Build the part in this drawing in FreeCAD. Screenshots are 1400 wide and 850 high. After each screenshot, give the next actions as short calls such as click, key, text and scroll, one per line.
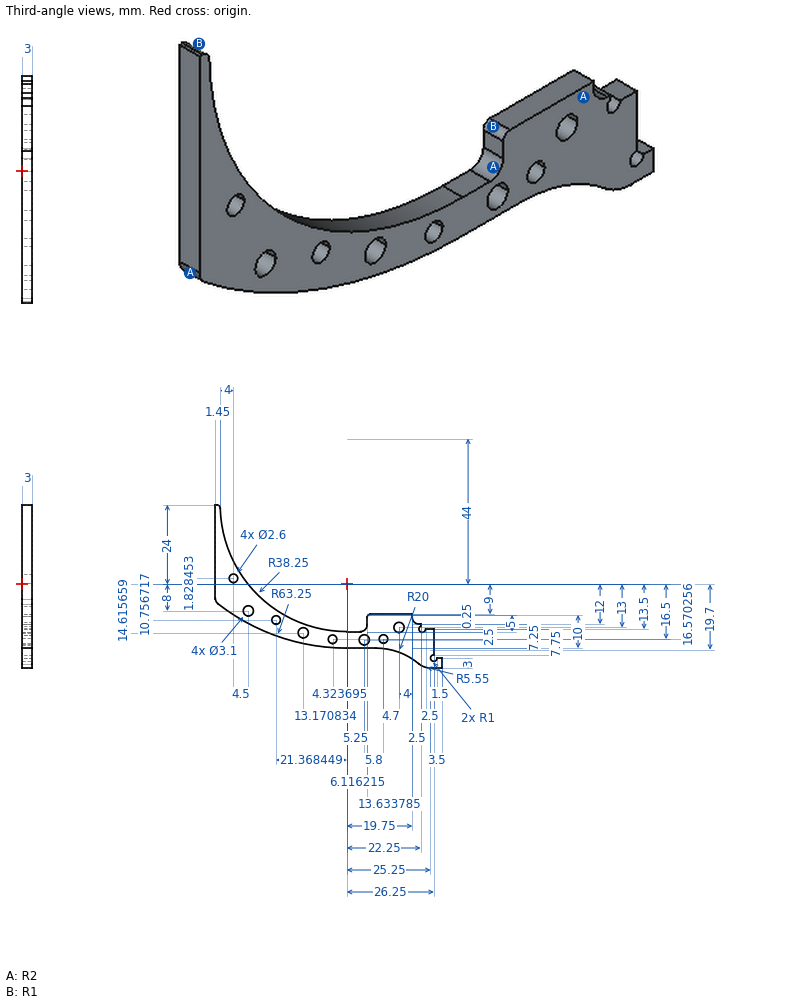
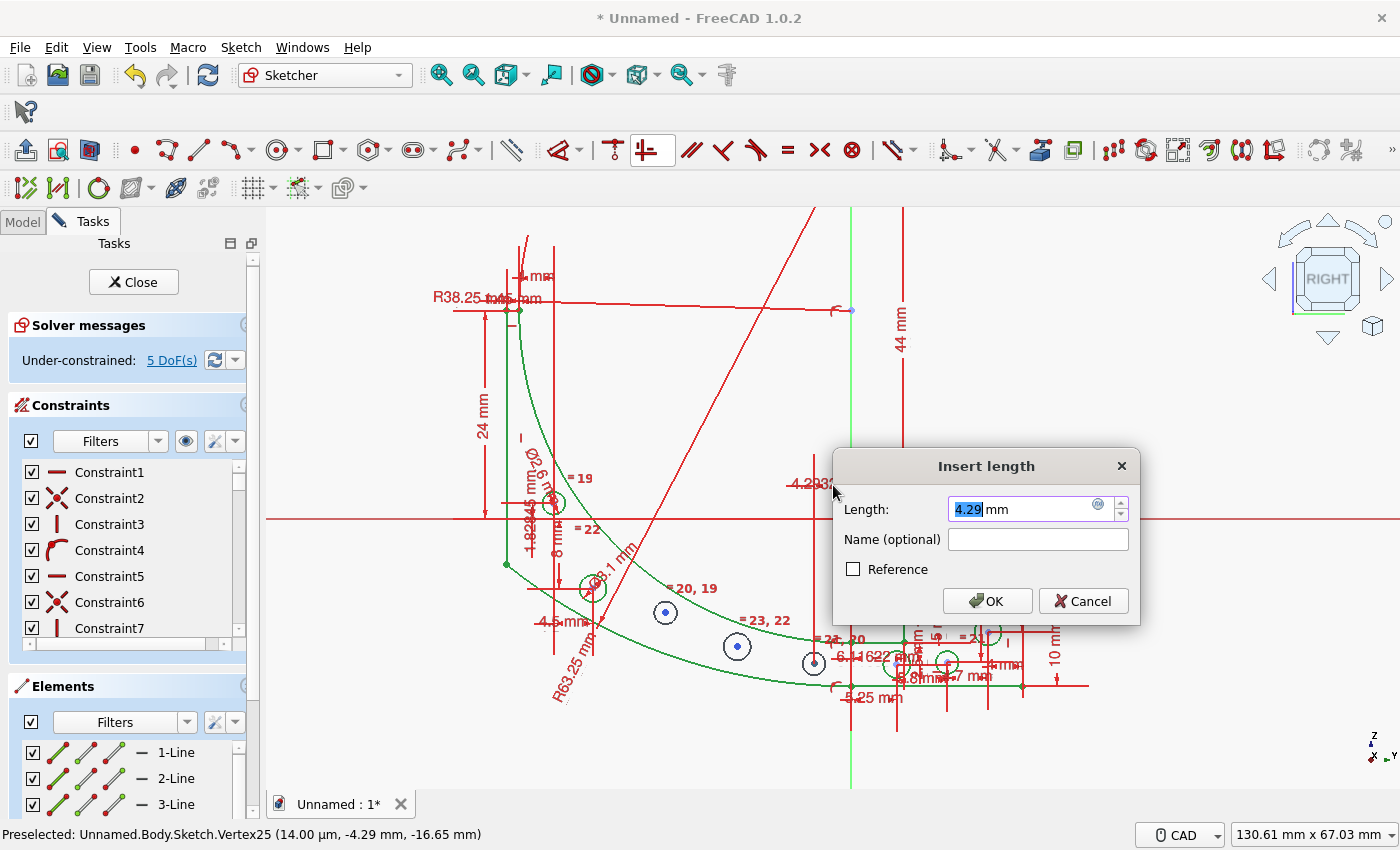
text(4.323695)
key(Return)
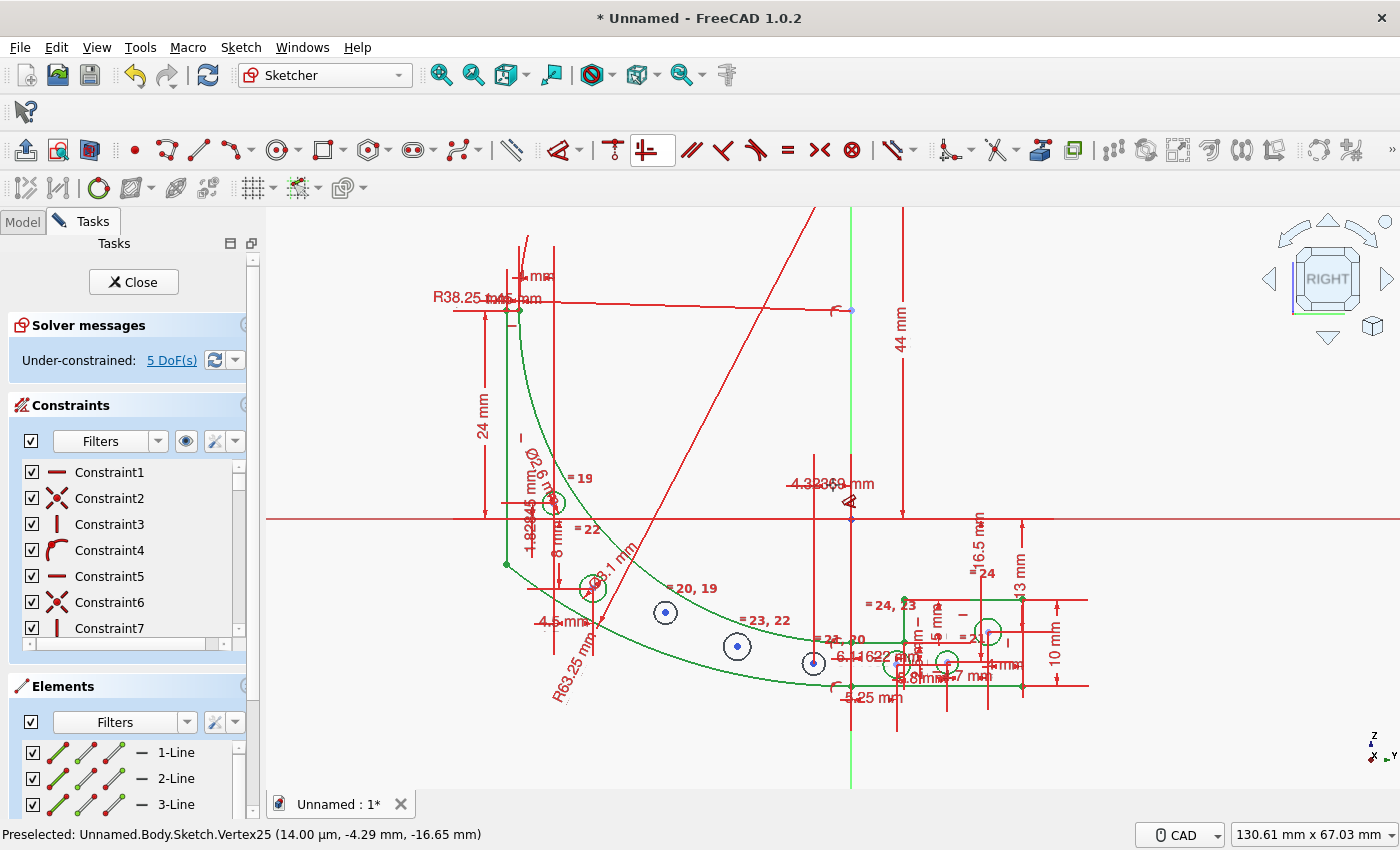
click(666, 613)
click(693, 647)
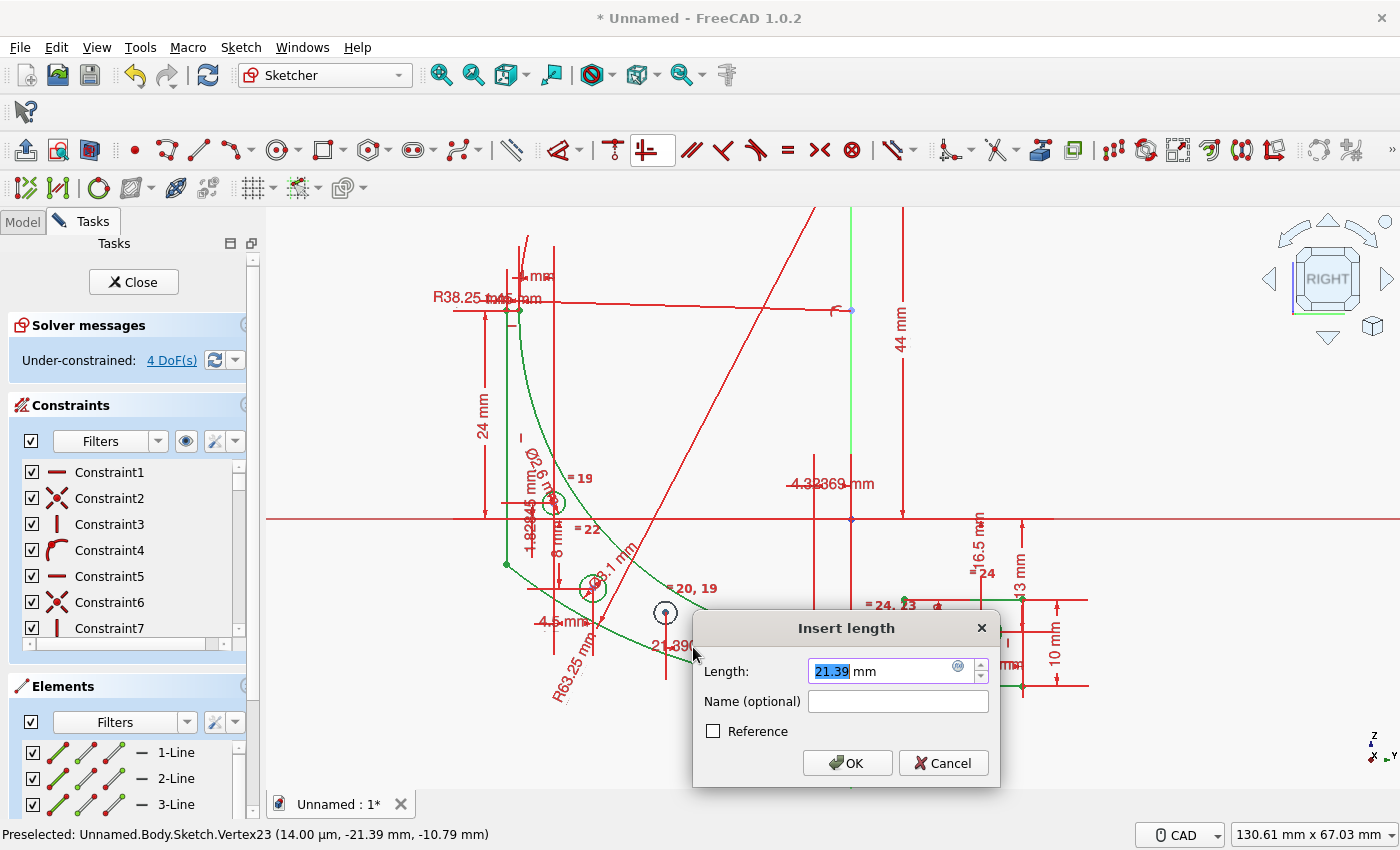
text(21.368449)
key(Return)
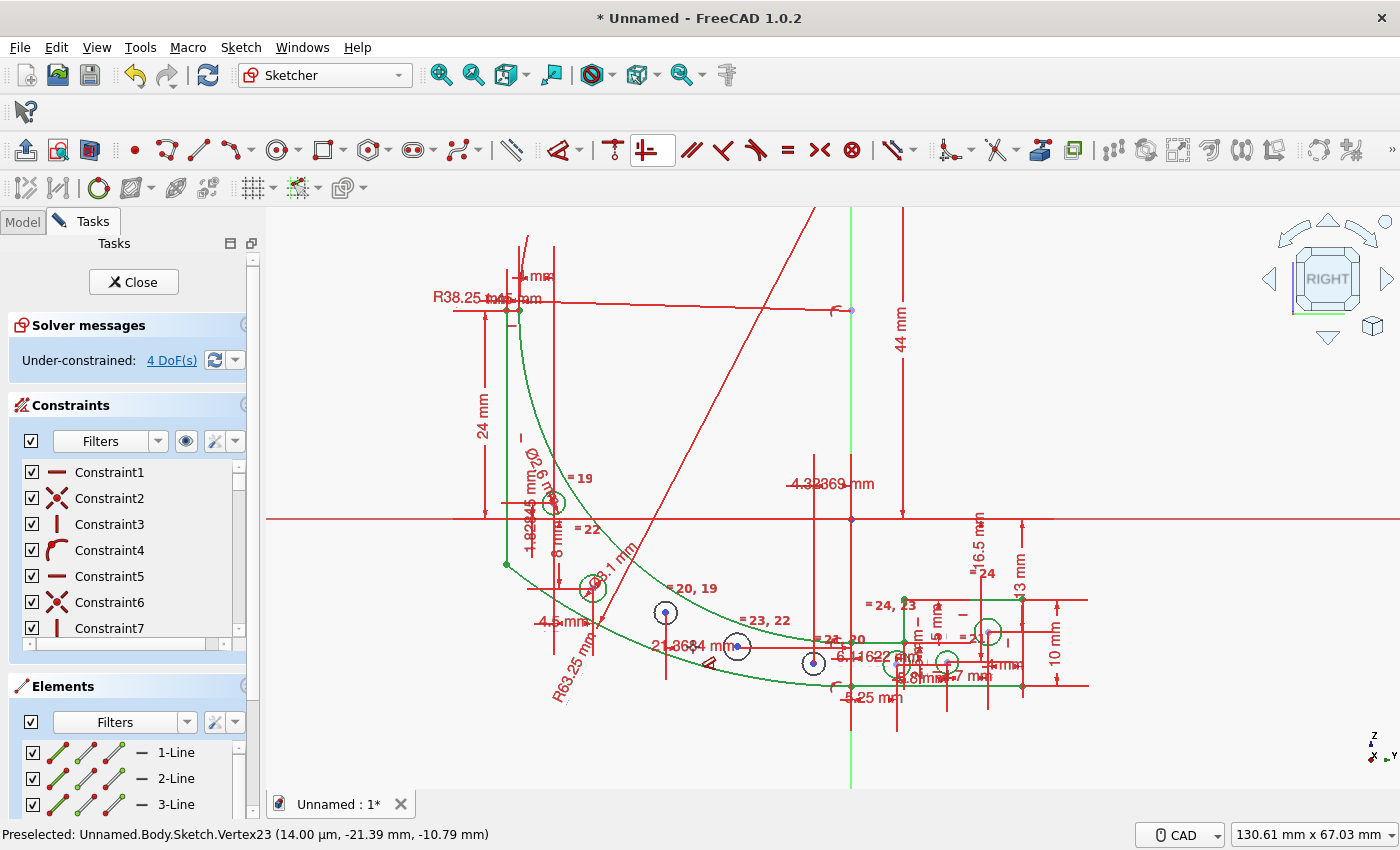
click(666, 613)
click(632, 588)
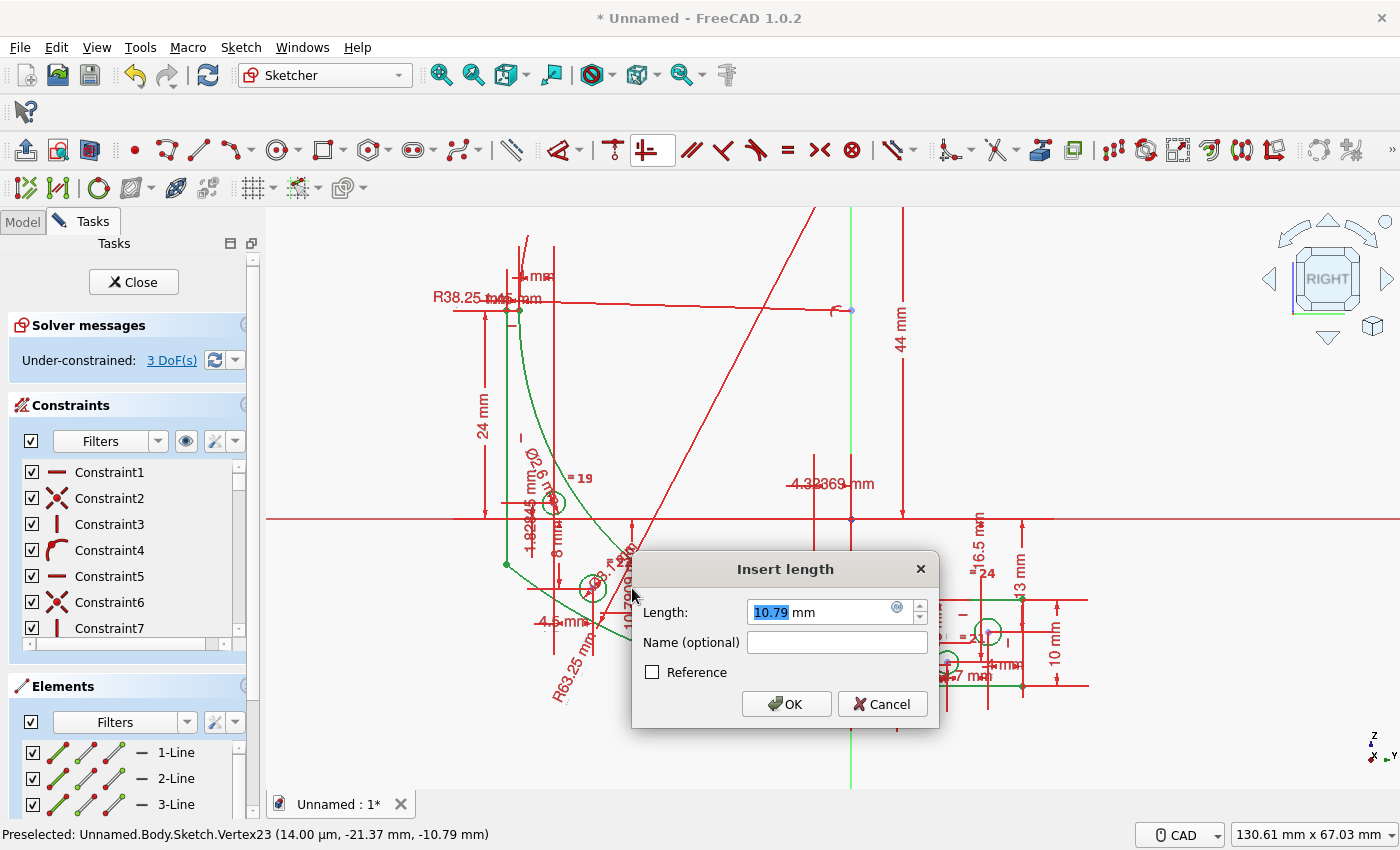
text(10.756717)
key(Return)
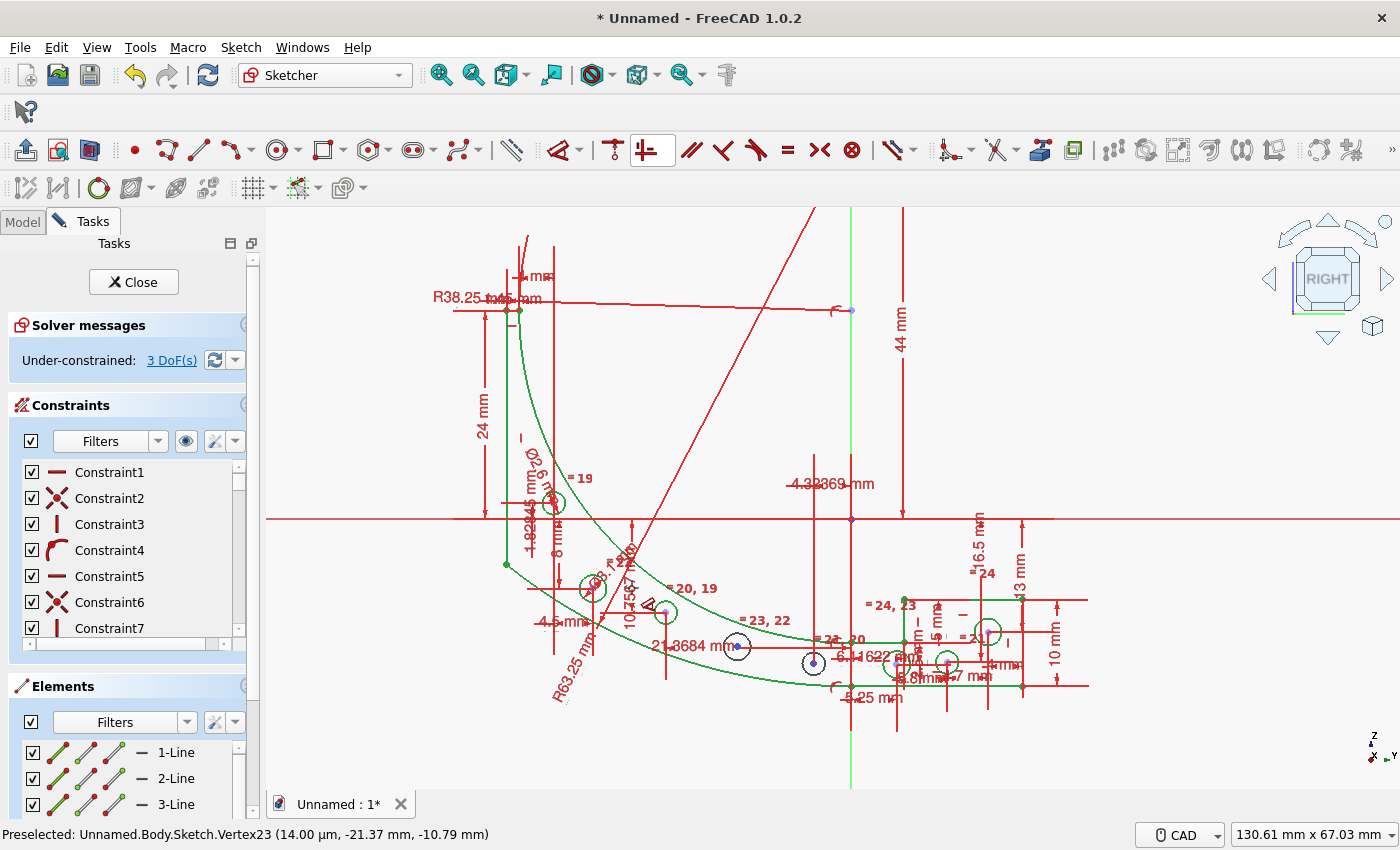
click(737, 647)
click(754, 485)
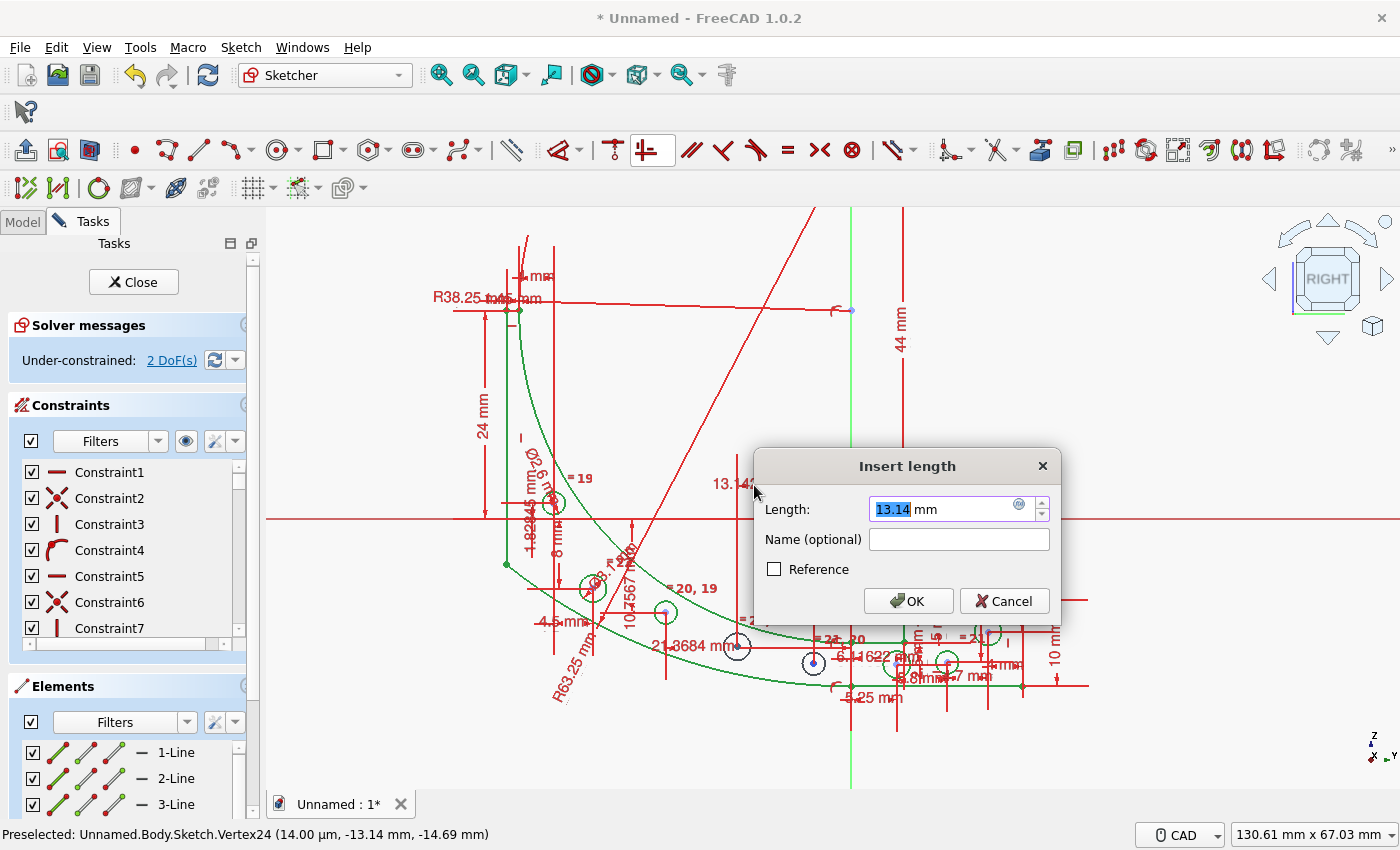
text(13.170834)
key(Return)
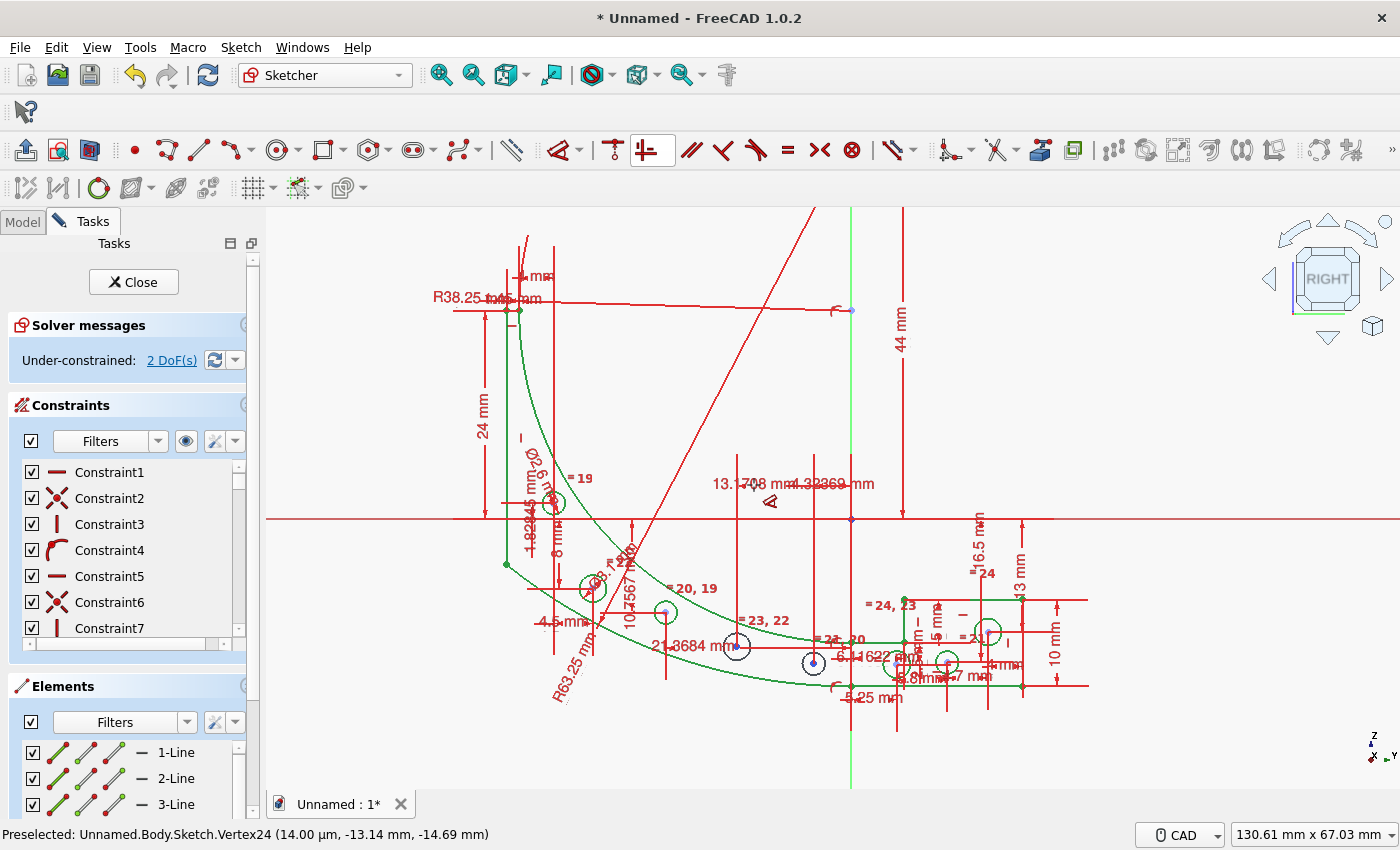
click(737, 647)
click(885, 583)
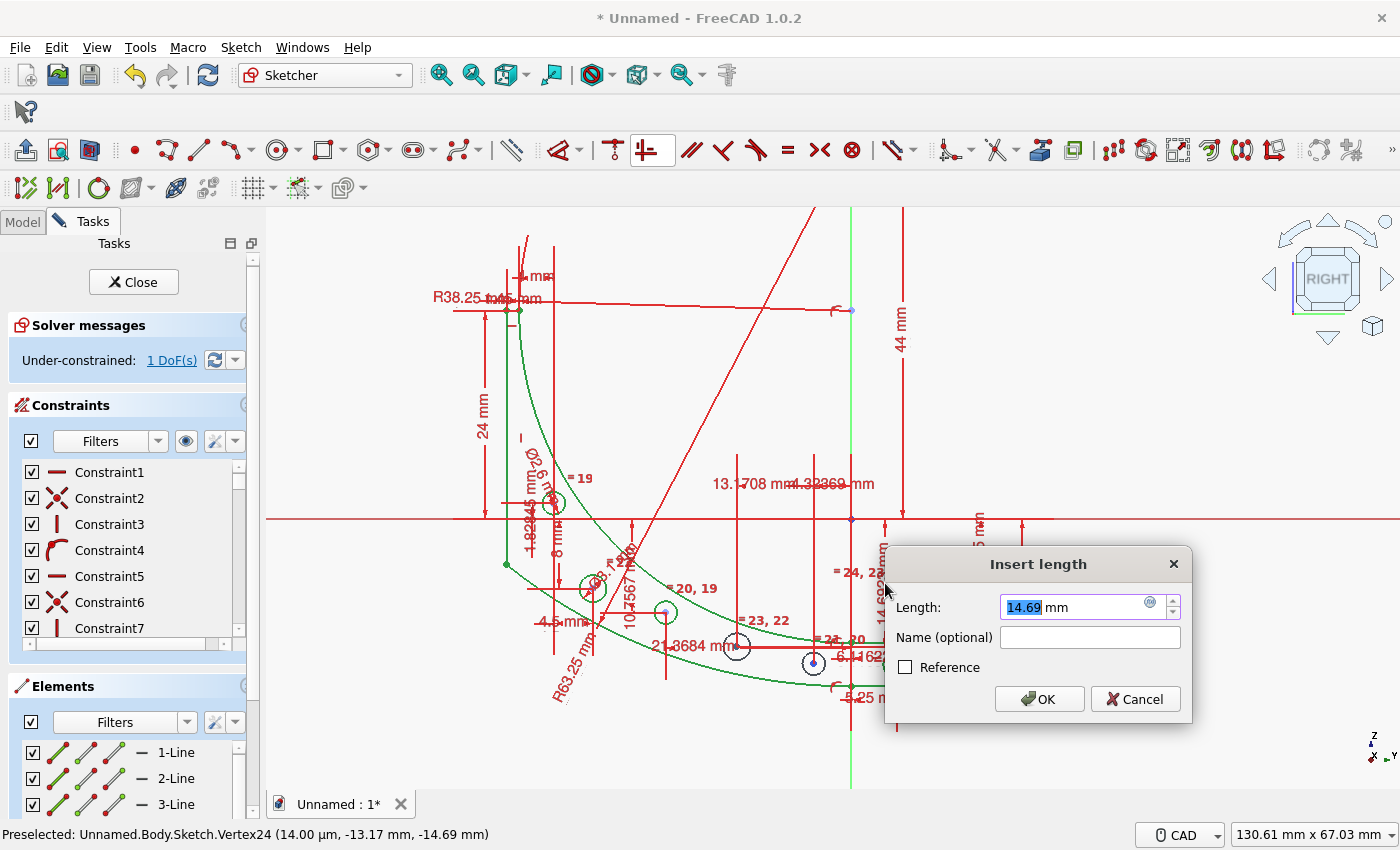
text(14.615659)
key(Return)